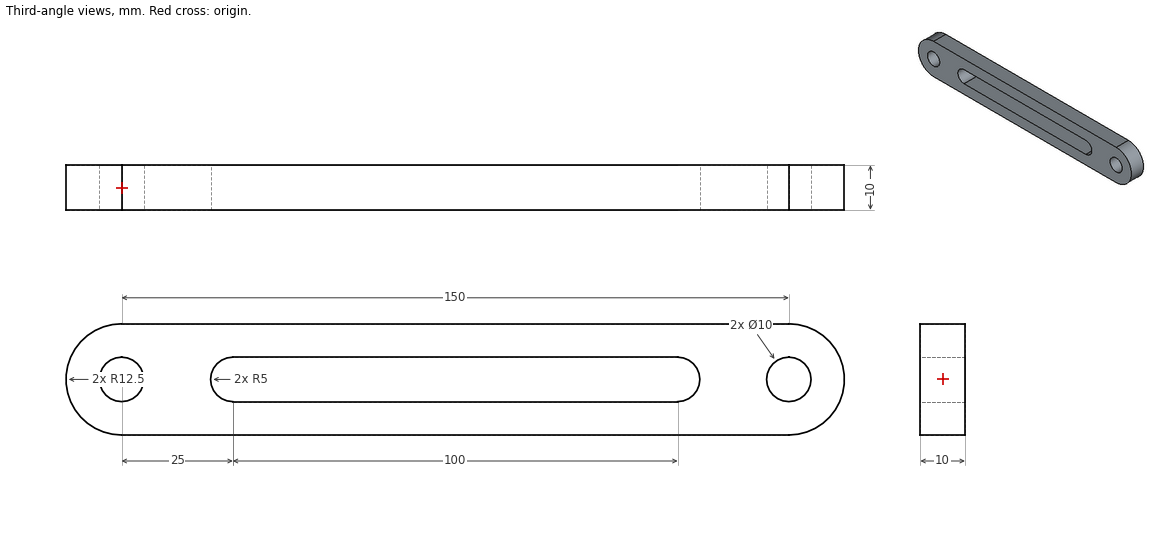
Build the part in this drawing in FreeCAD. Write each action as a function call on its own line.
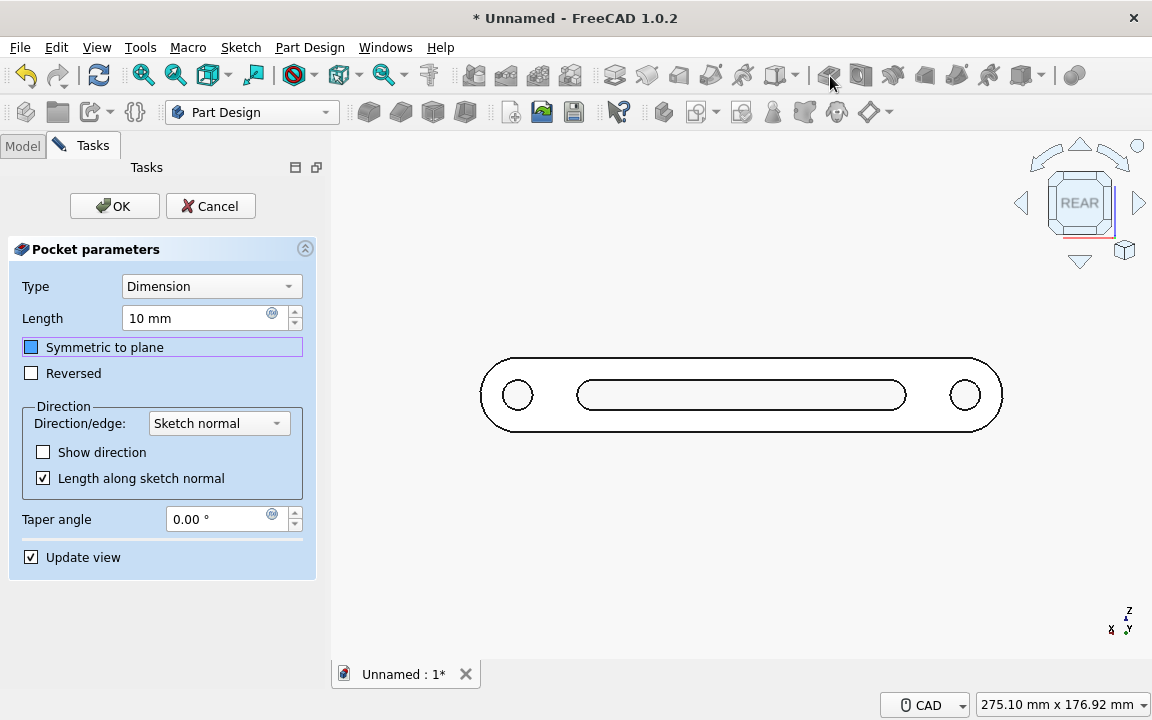
click(115, 206)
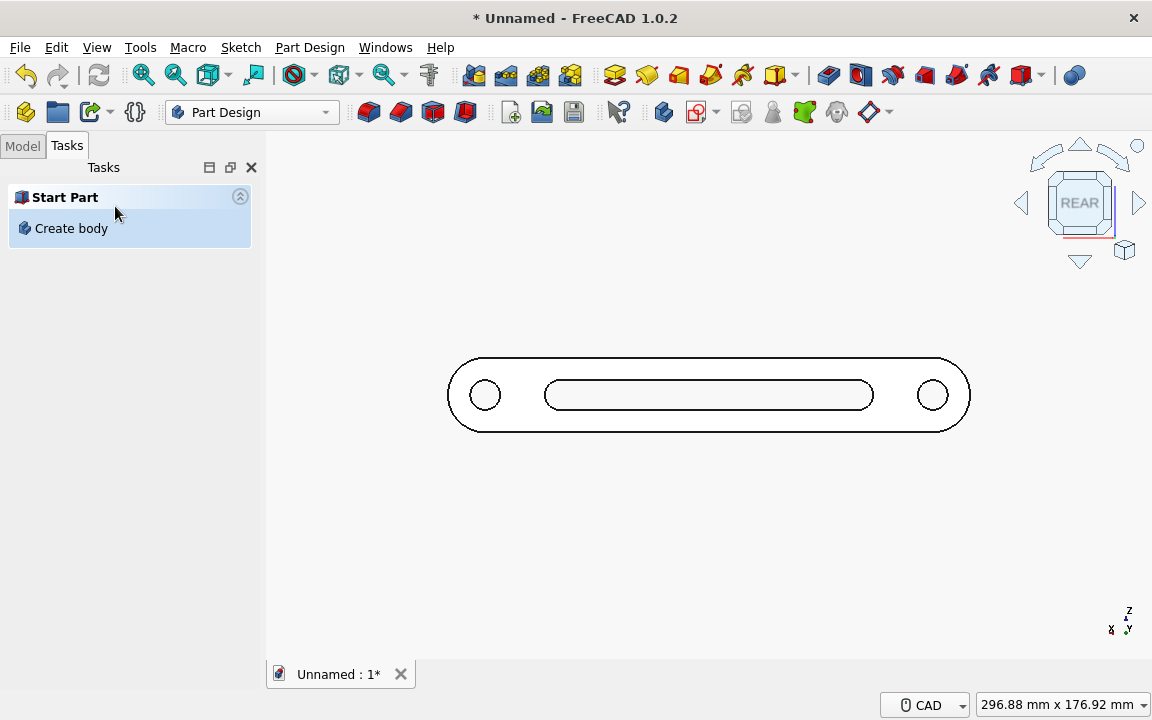
key(0)